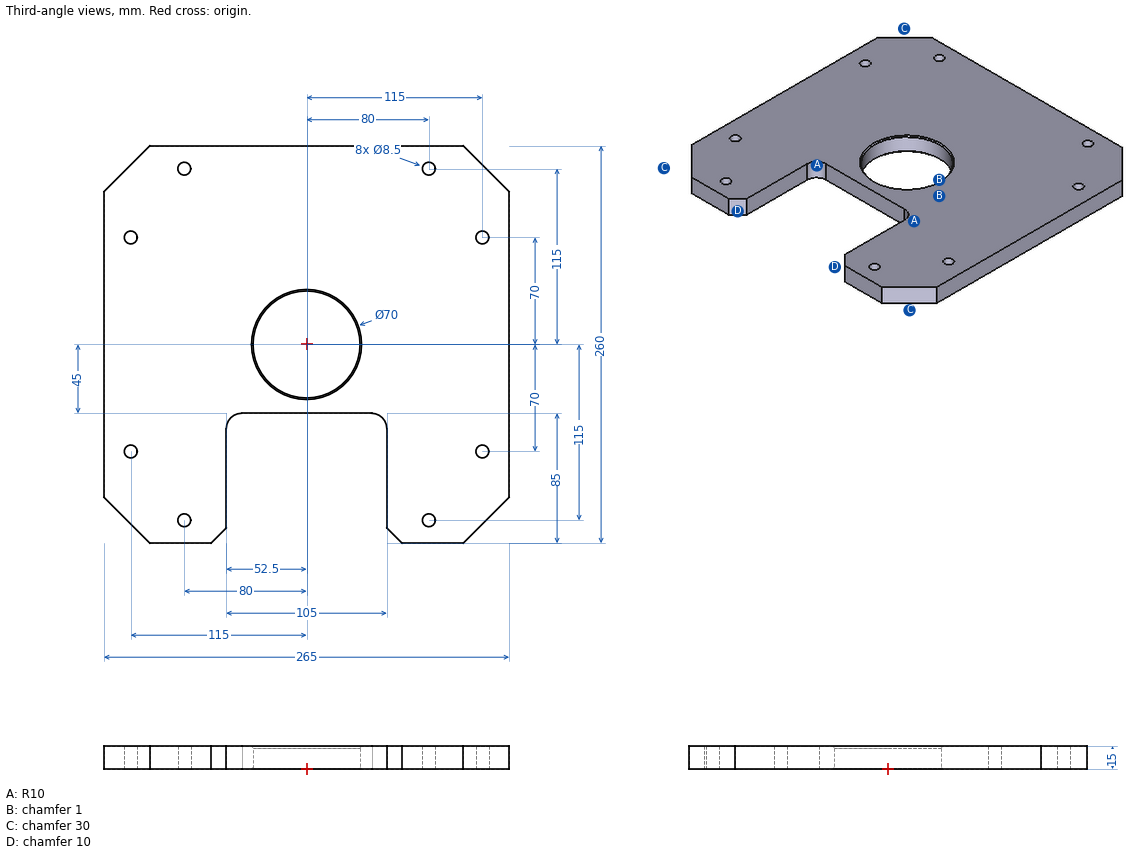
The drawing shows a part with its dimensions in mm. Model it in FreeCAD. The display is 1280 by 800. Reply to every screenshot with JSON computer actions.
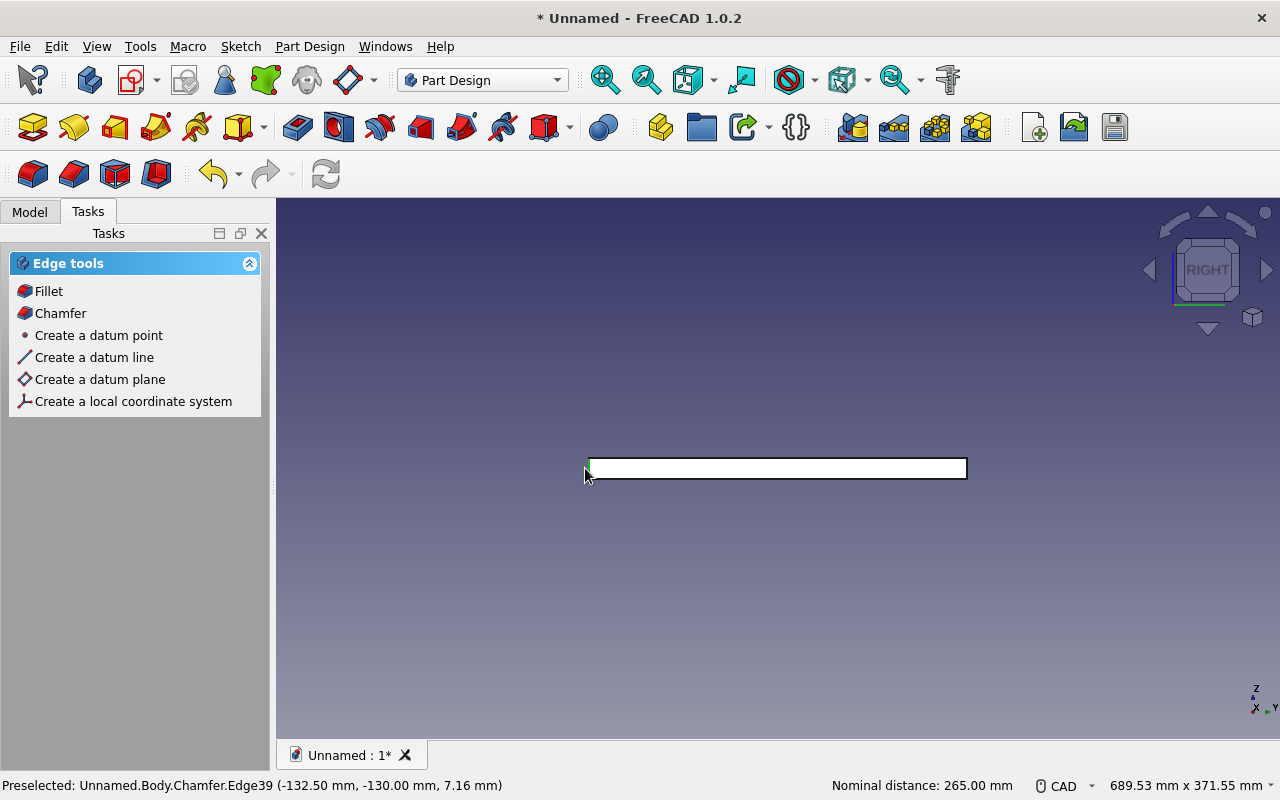
{"action": "key", "text": "v f"}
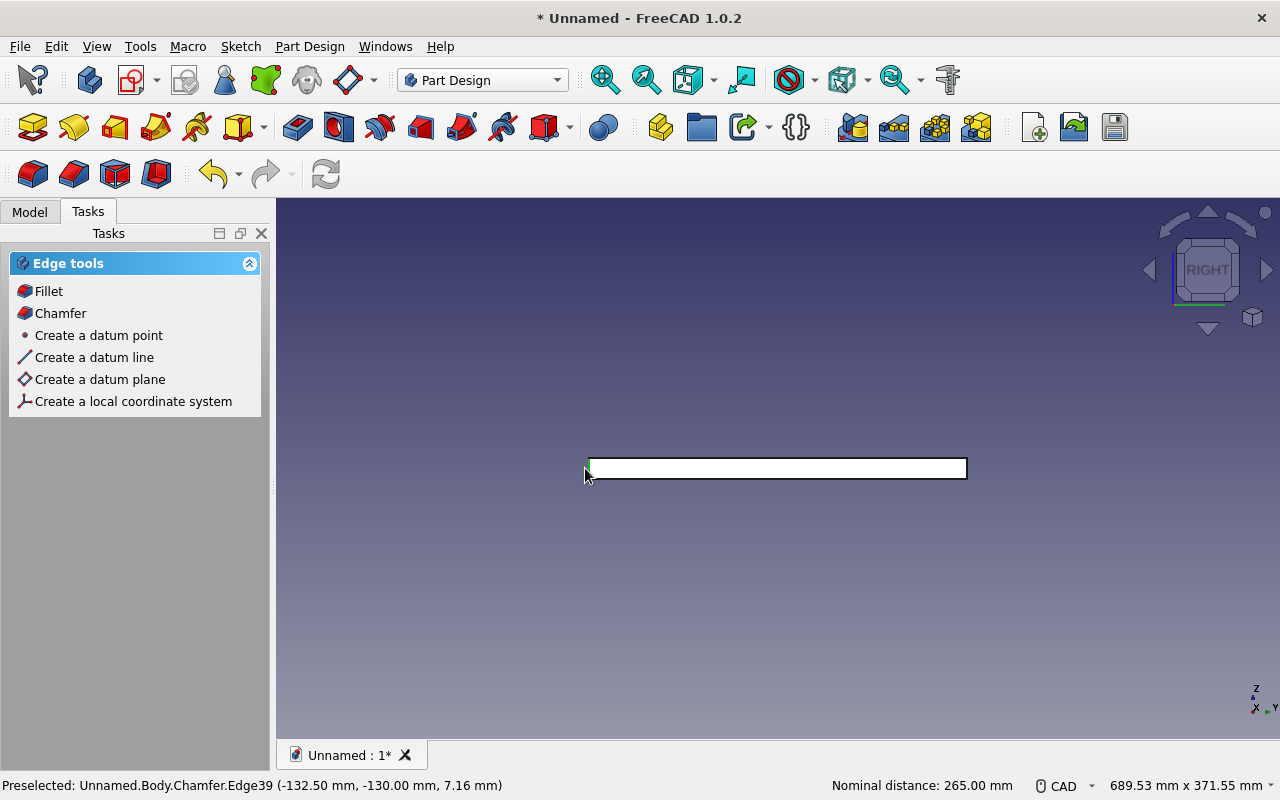
{"action": "left_click", "coordinate": [967, 467], "text": "ctrl"}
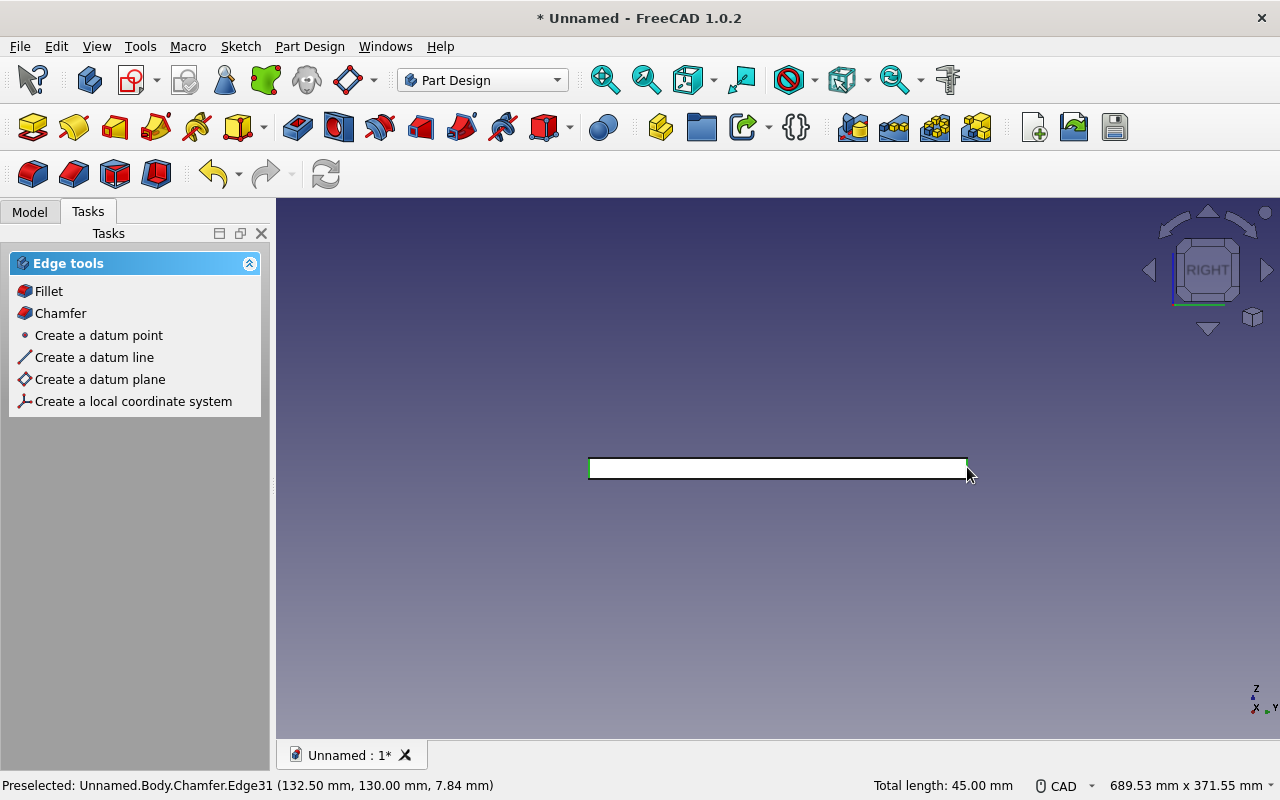
{"action": "scroll", "coordinate": [967, 467], "scroll_direction": "up", "scroll_amount": 4}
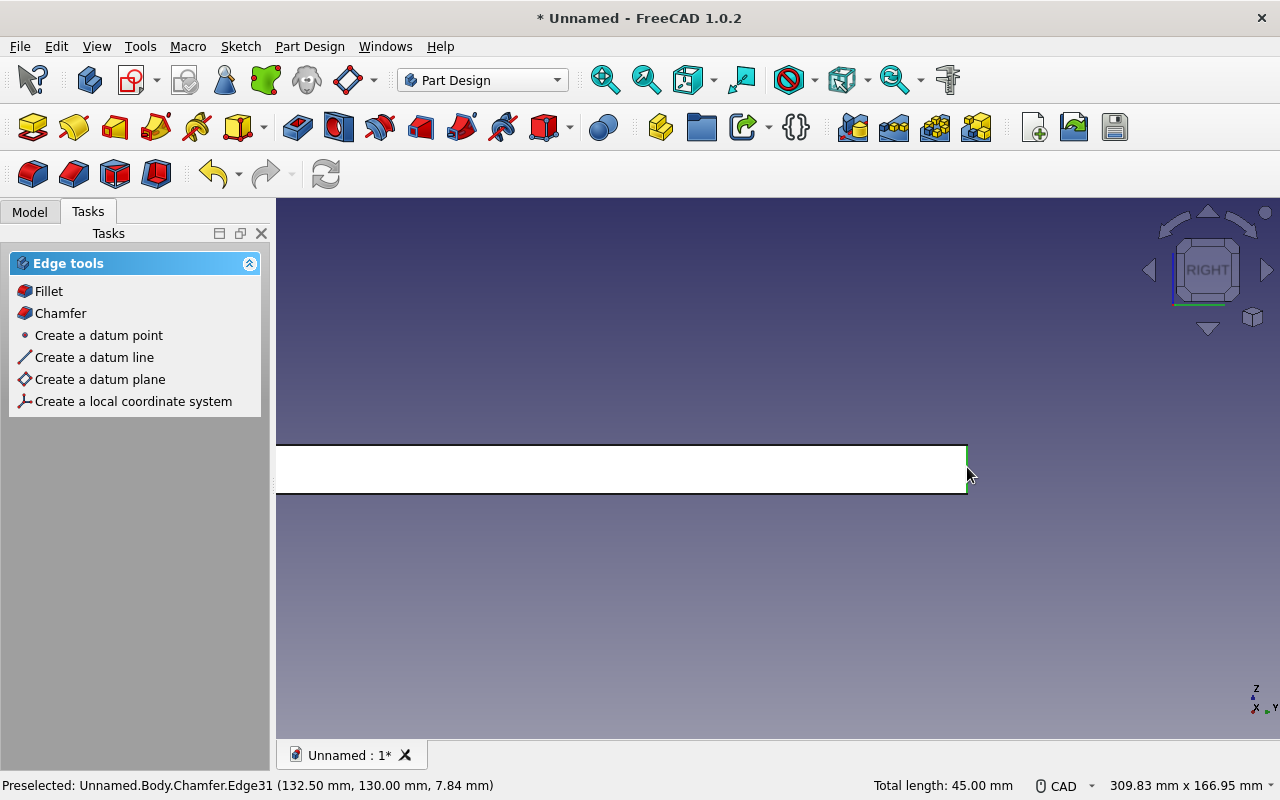
{"action": "key", "text": "v f"}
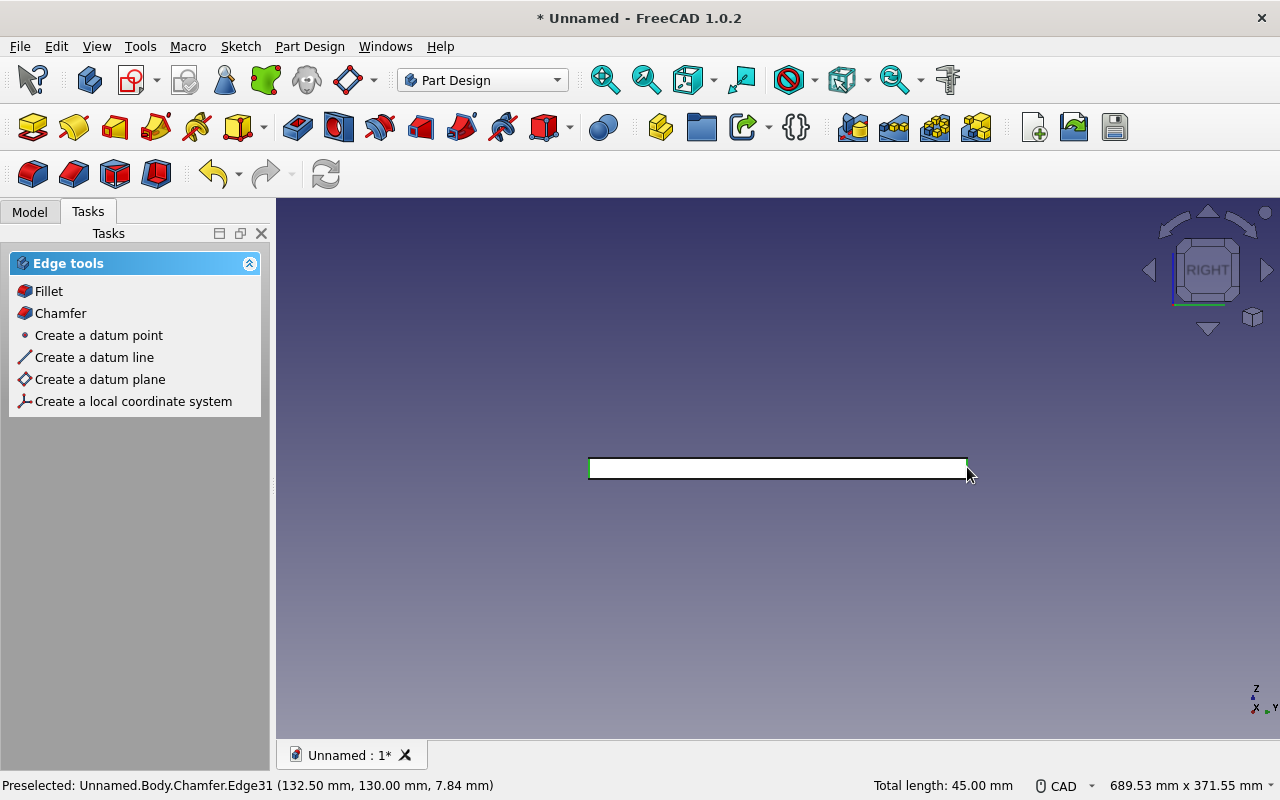
{"action": "key", "text": "5"}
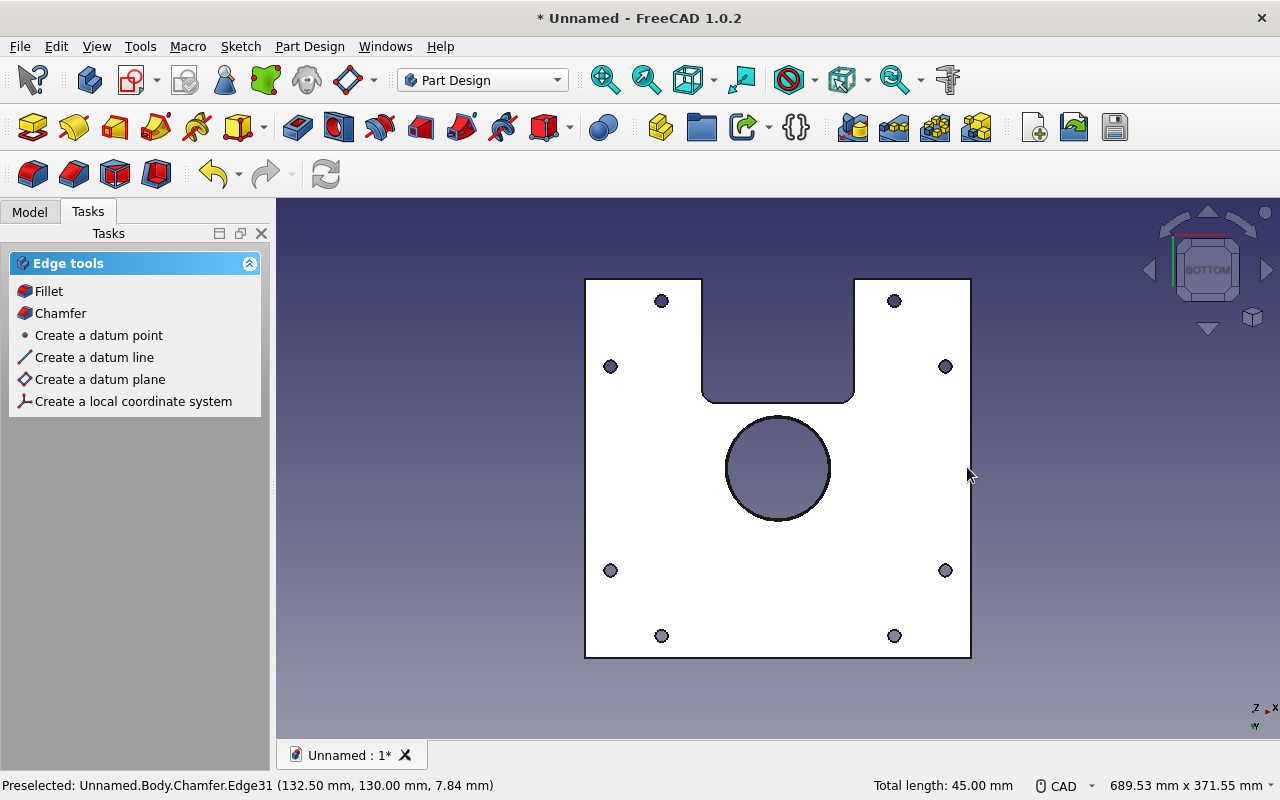
{"action": "scroll", "coordinate": [585, 657], "scroll_direction": "up", "scroll_amount": 4}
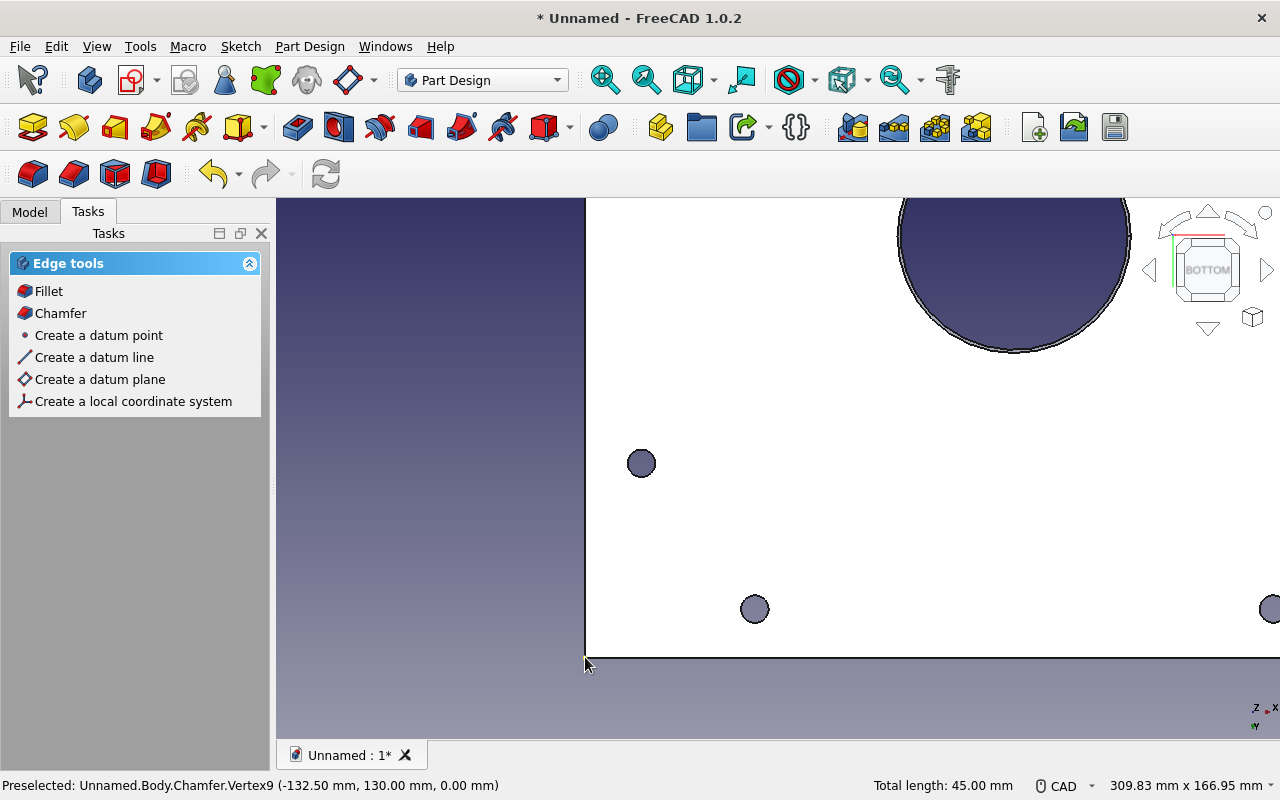
{"action": "left_click", "coordinate": [606, 80]}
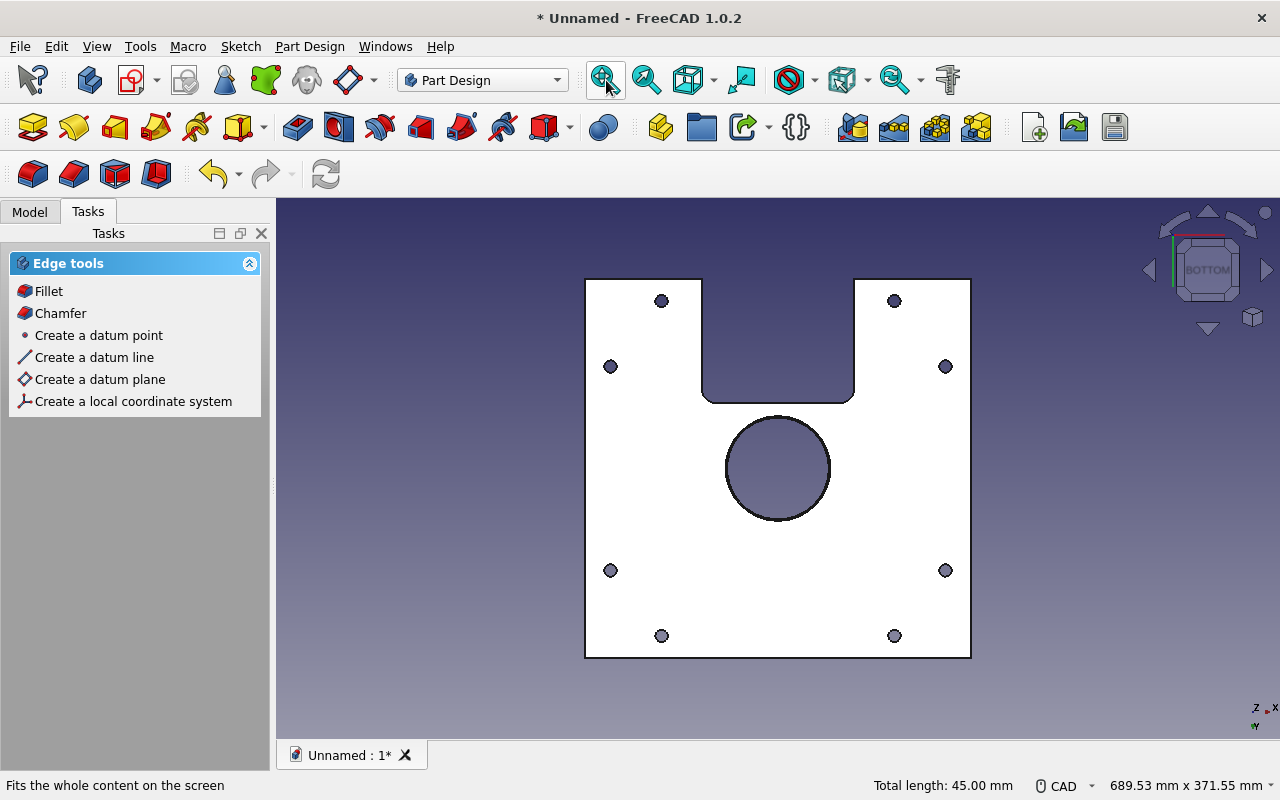
{"action": "key", "text": "4"}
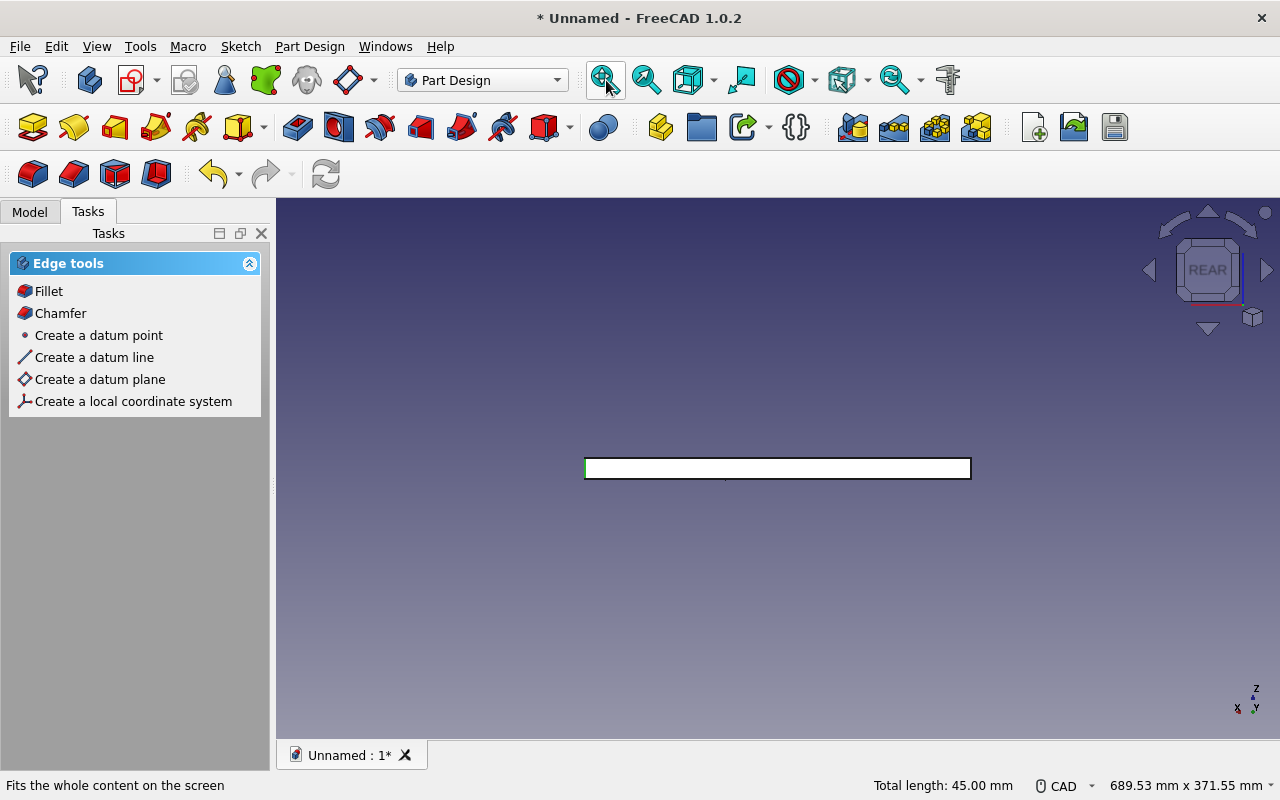
{"action": "left_click", "coordinate": [606, 80]}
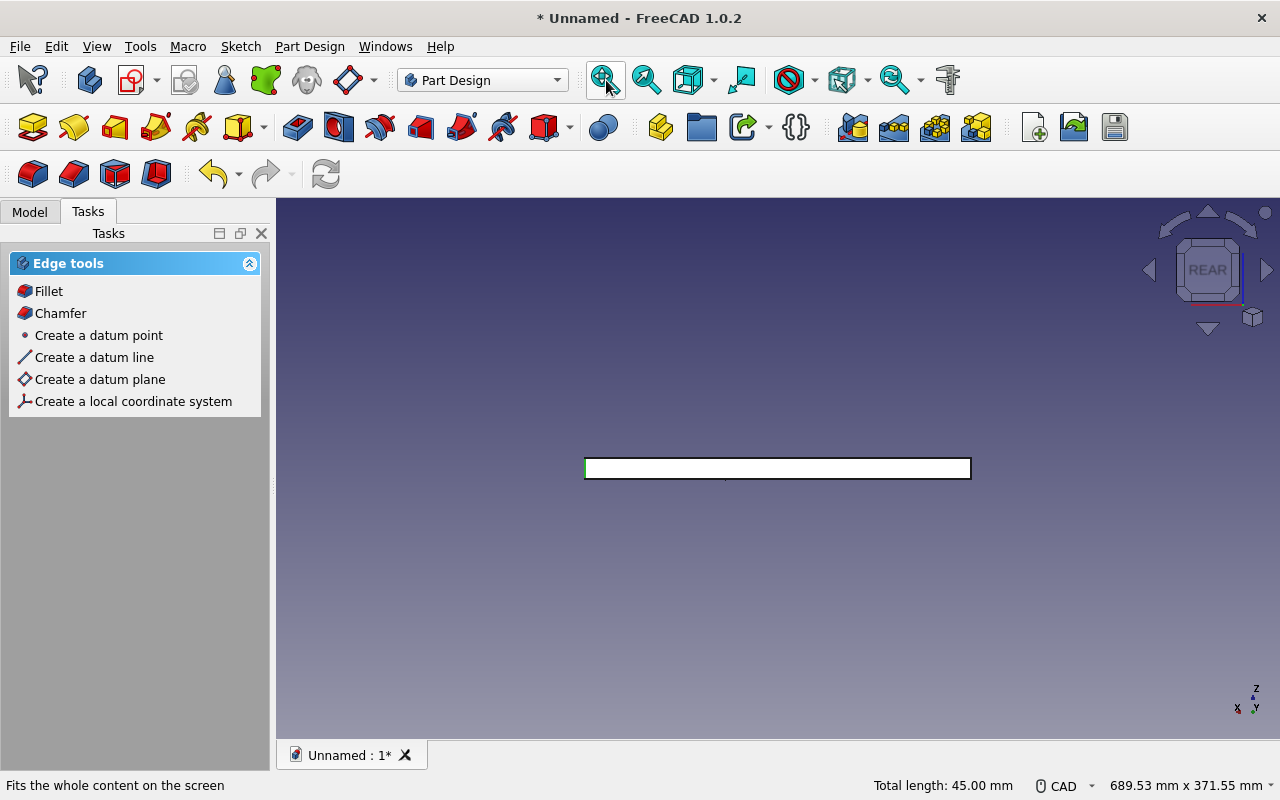
{"action": "left_click", "coordinate": [971, 468], "text": "ctrl"}